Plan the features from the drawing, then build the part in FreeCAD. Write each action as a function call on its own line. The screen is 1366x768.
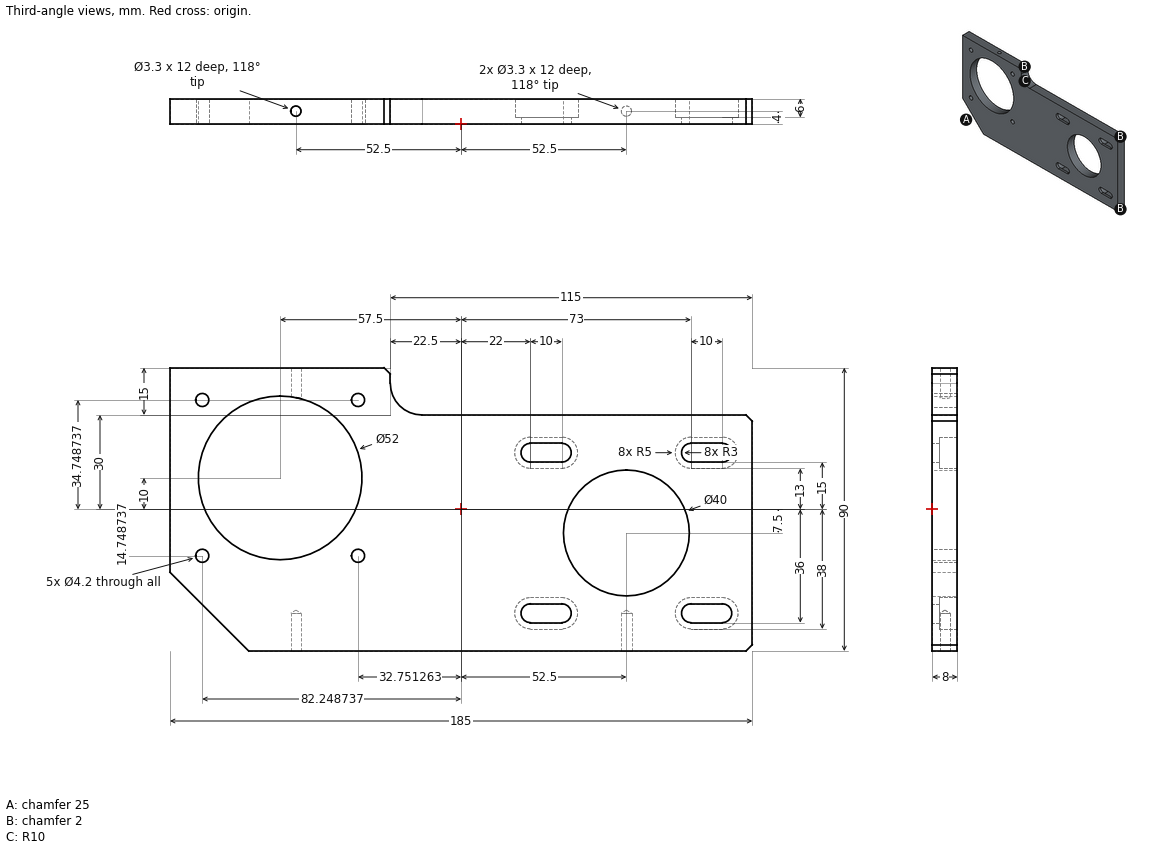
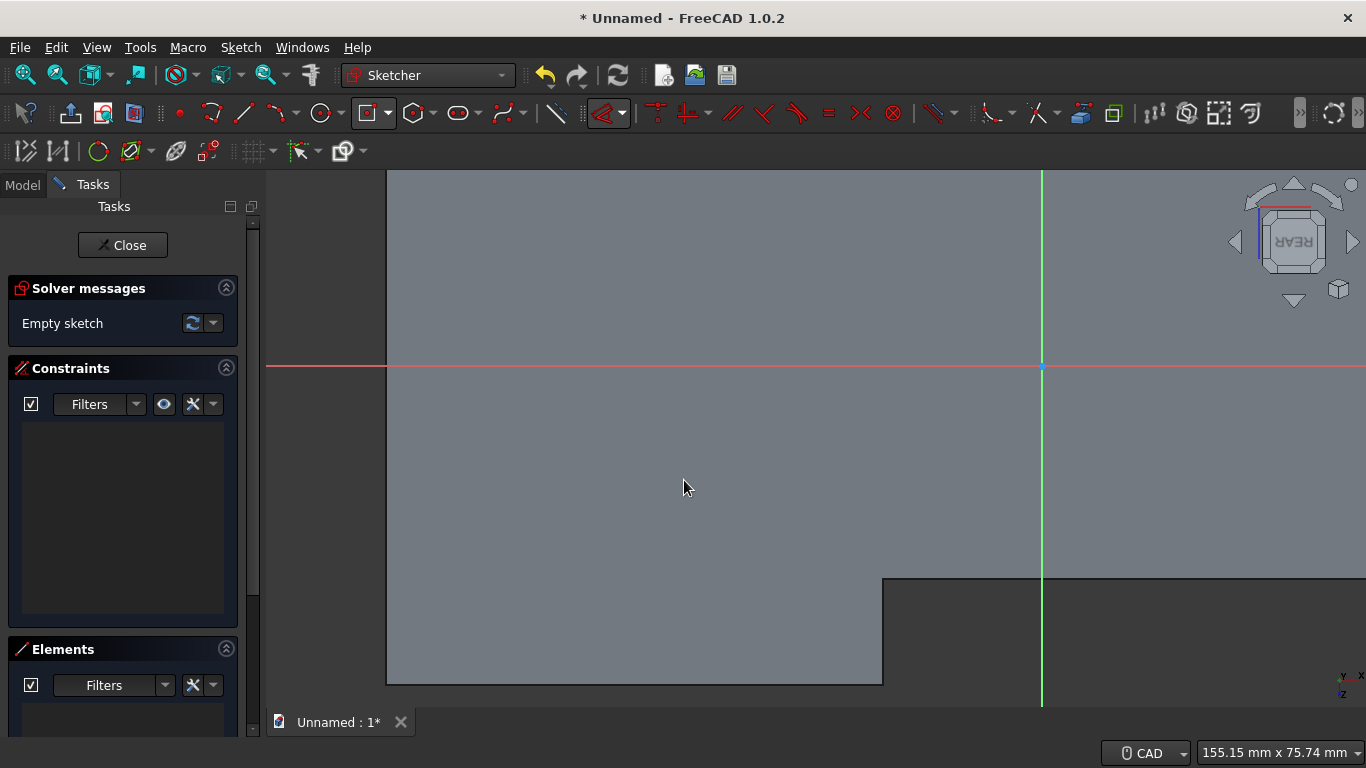
click(322, 114)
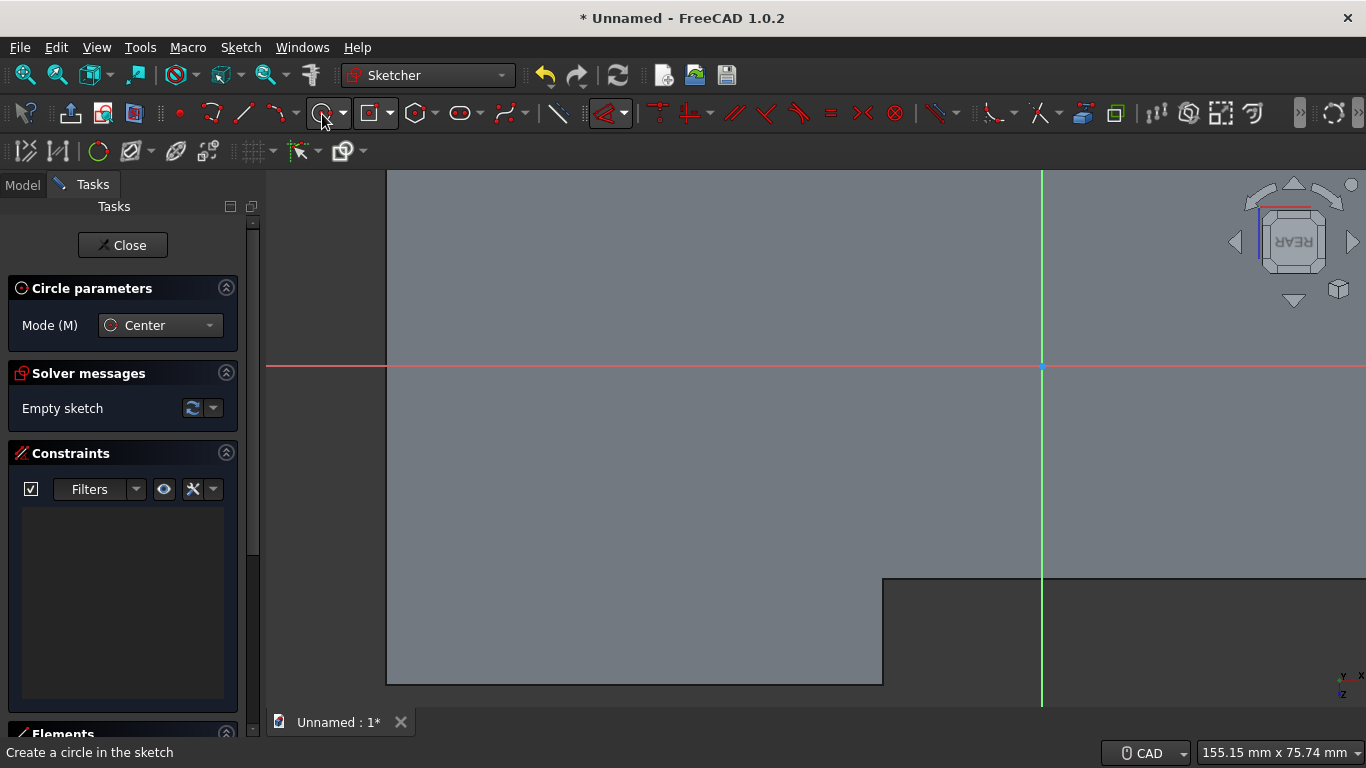
click(634, 437)
click(765, 307)
key(Escape)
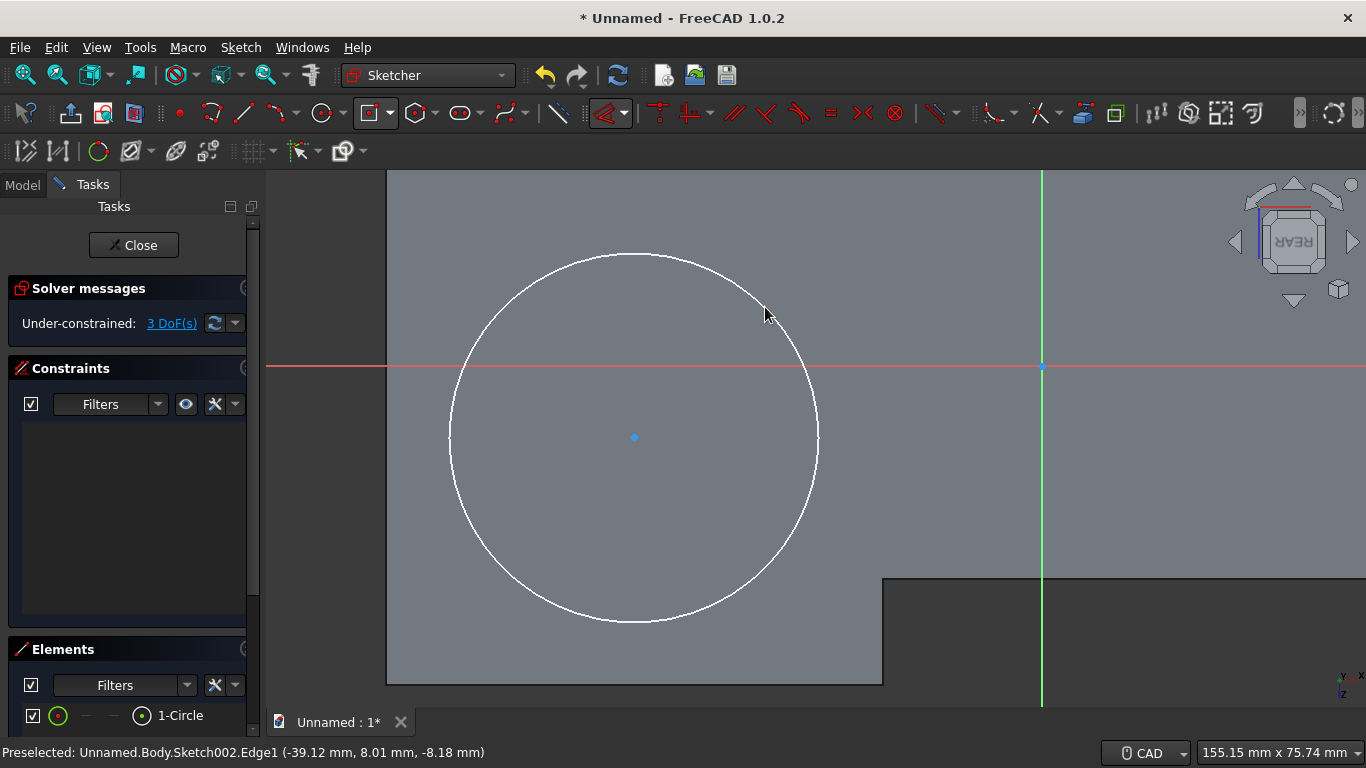
click(764, 307)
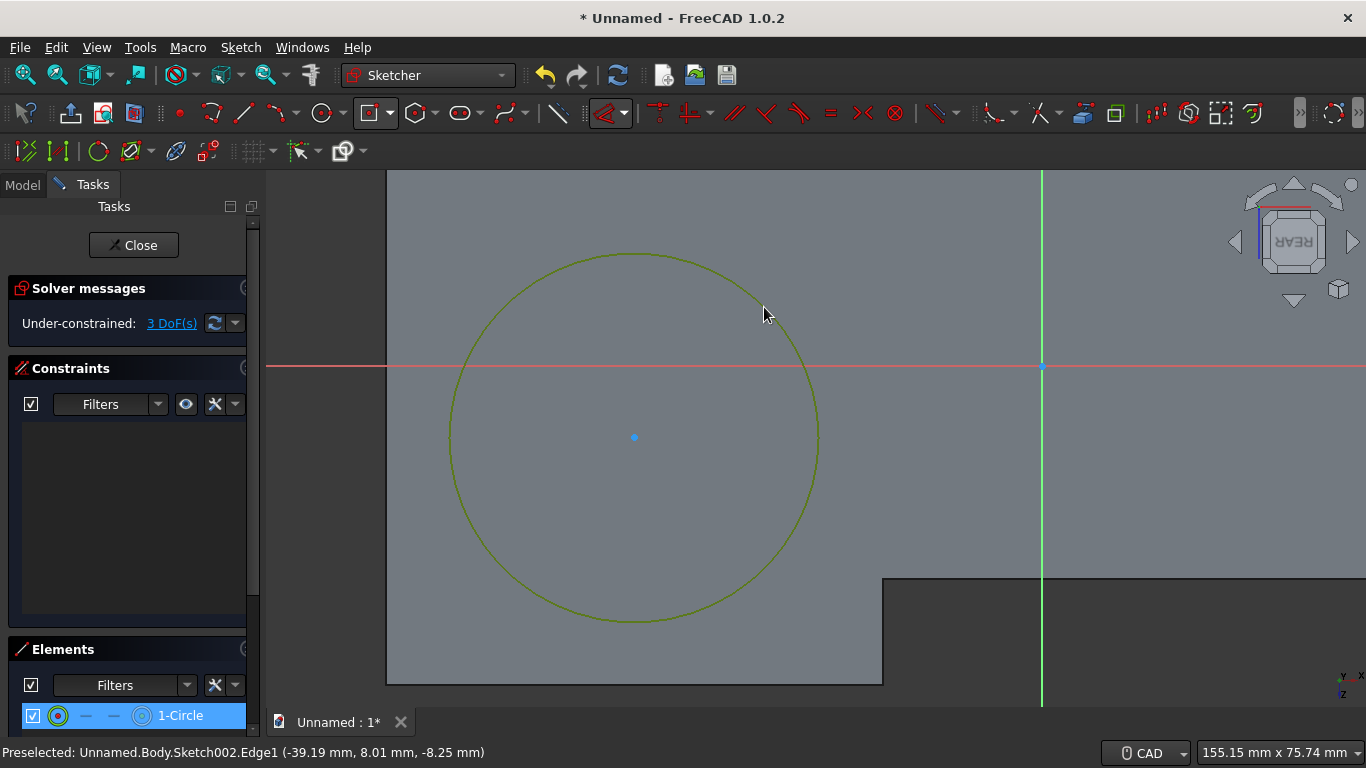
key(k)
key(o)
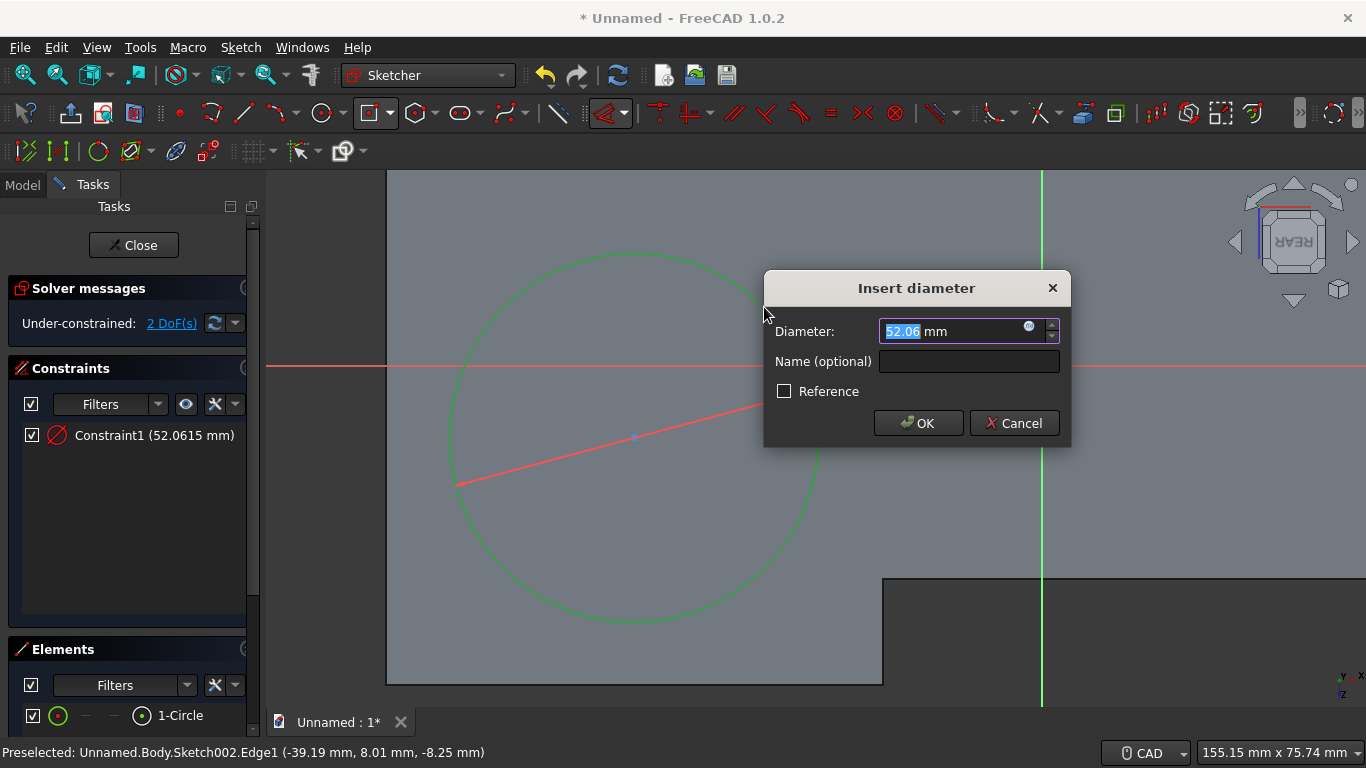
text(52)
key(Return)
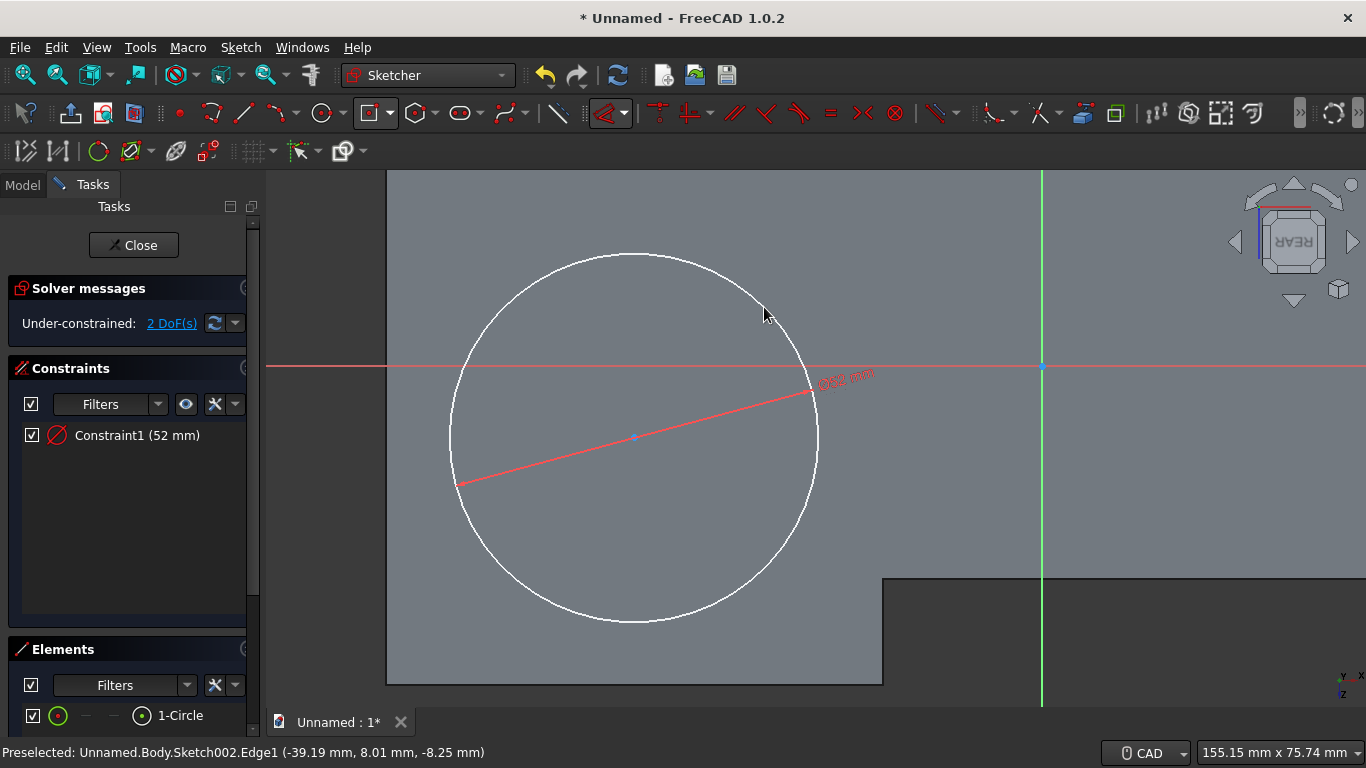
click(634, 438)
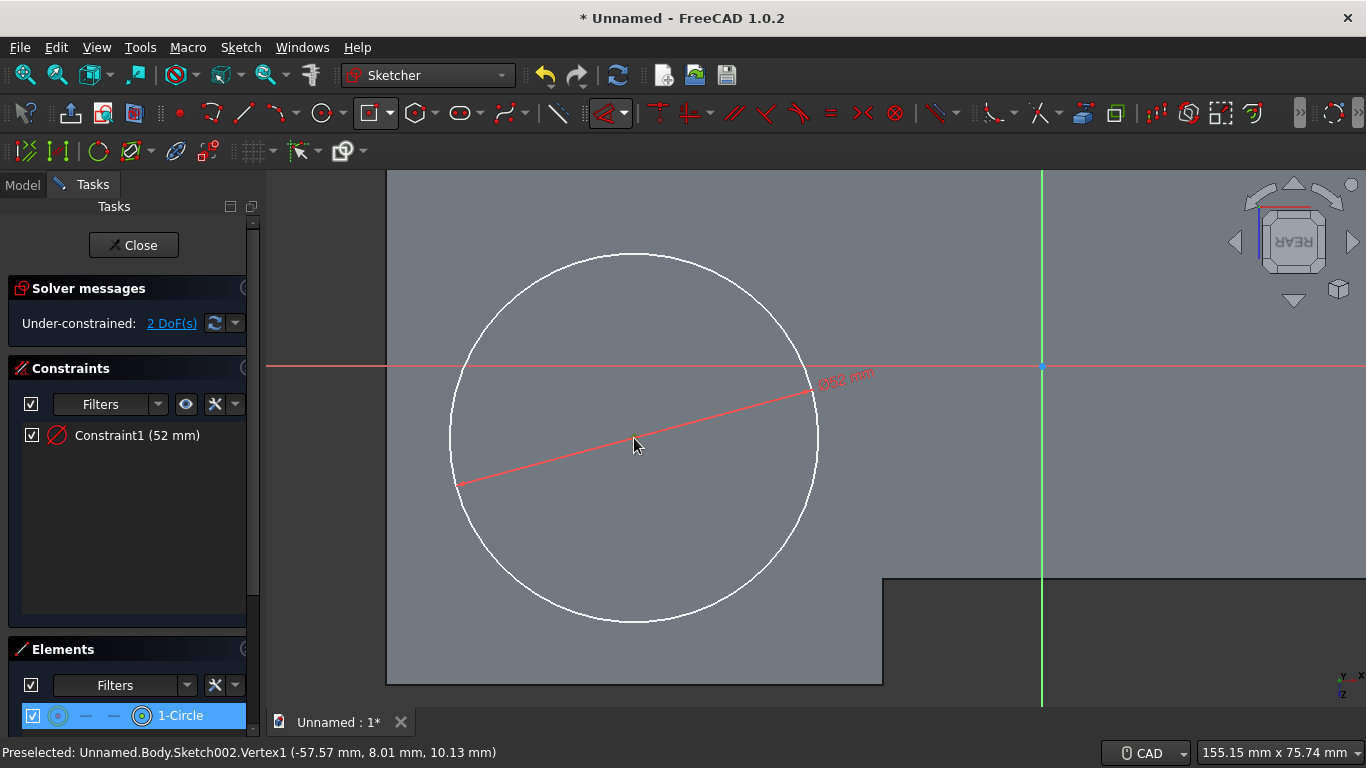
key(i)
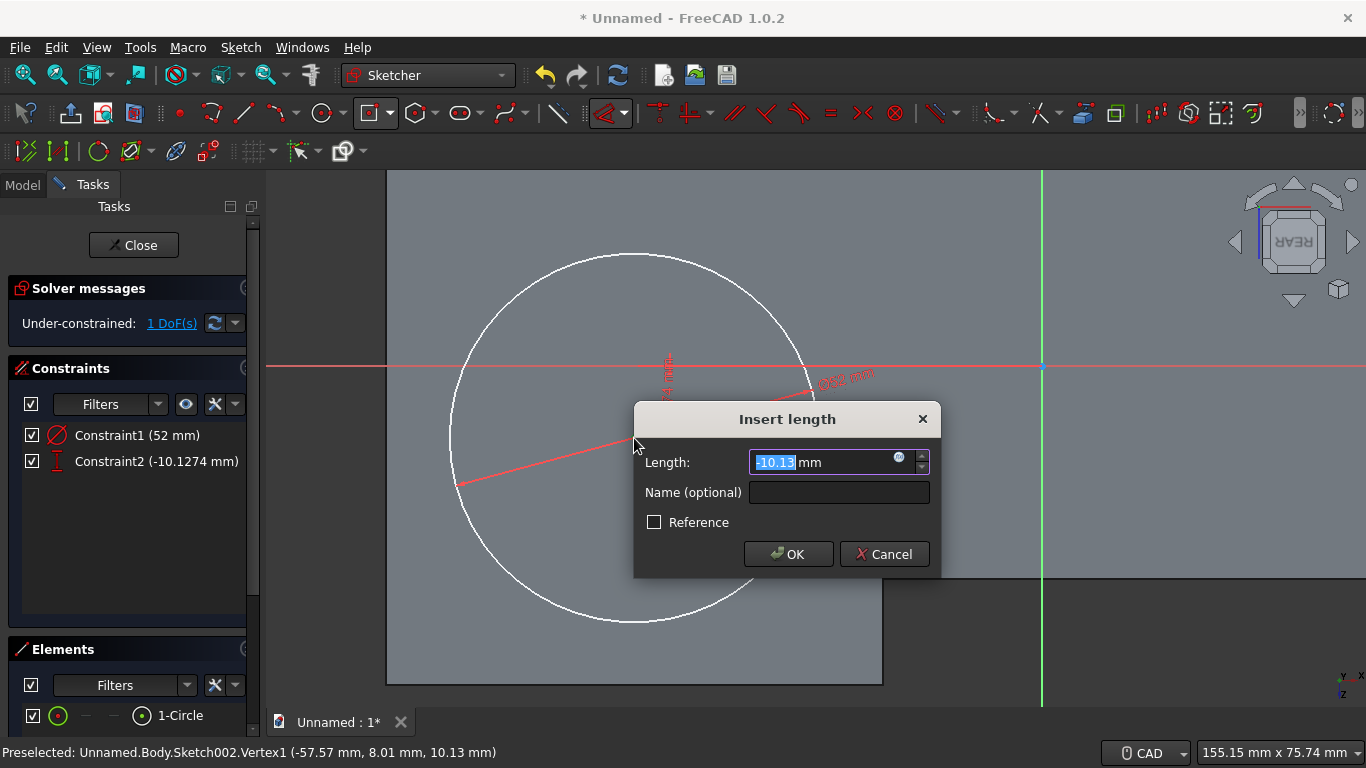
text(-10)
key(Return)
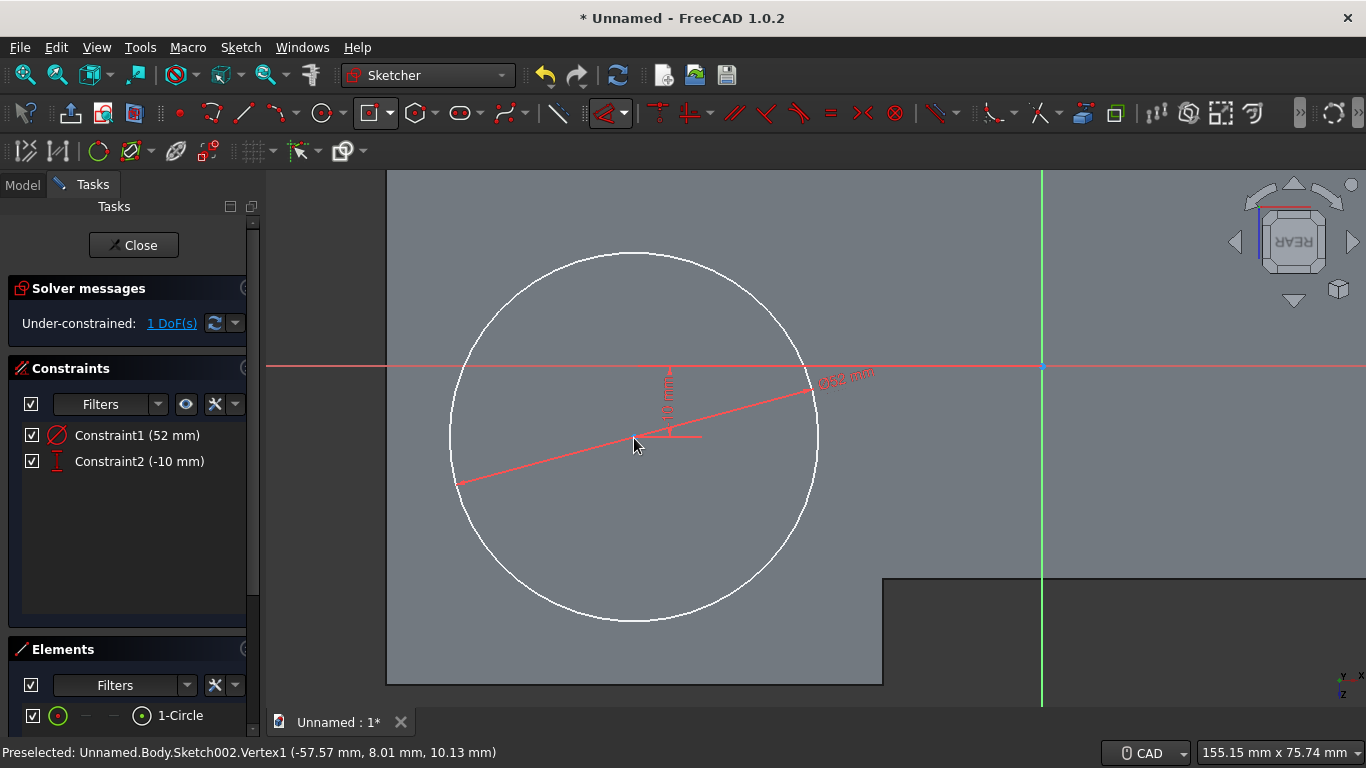
click(634, 437)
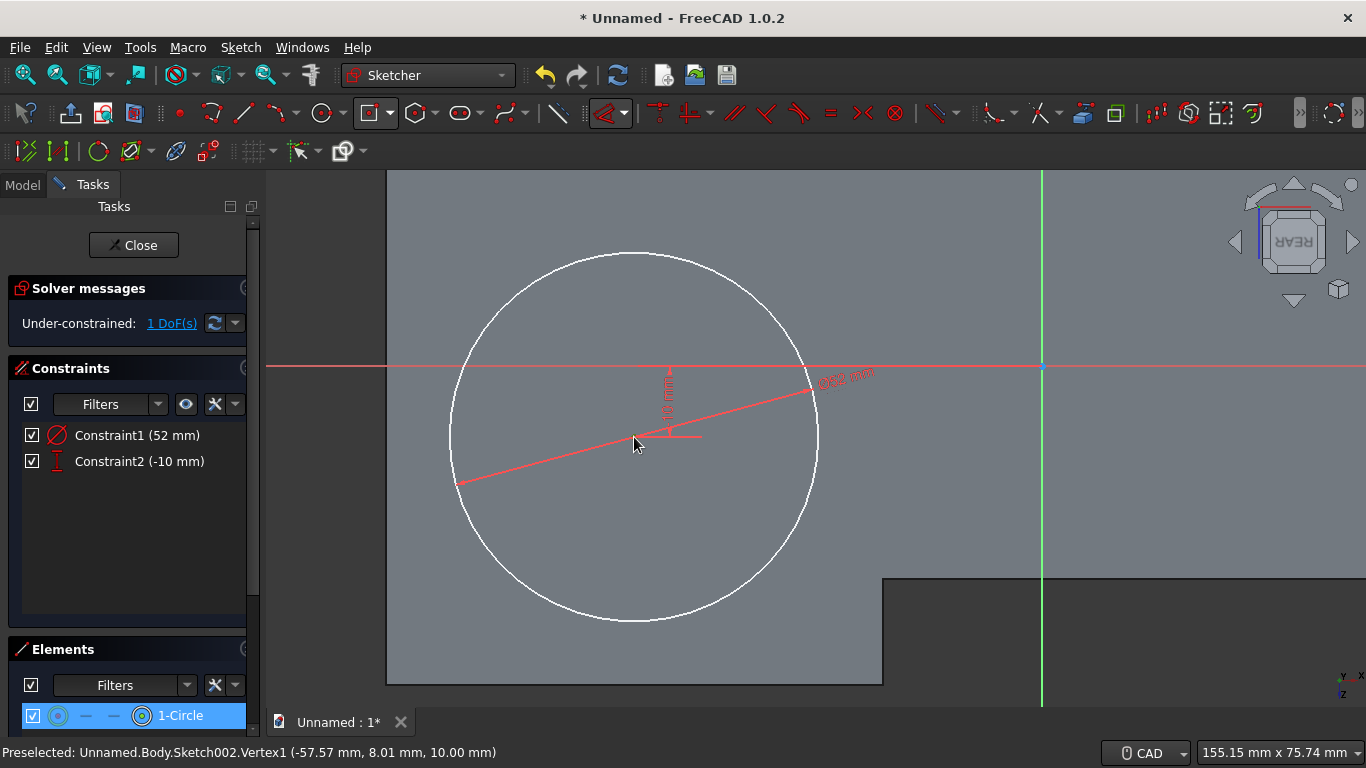
key(l)